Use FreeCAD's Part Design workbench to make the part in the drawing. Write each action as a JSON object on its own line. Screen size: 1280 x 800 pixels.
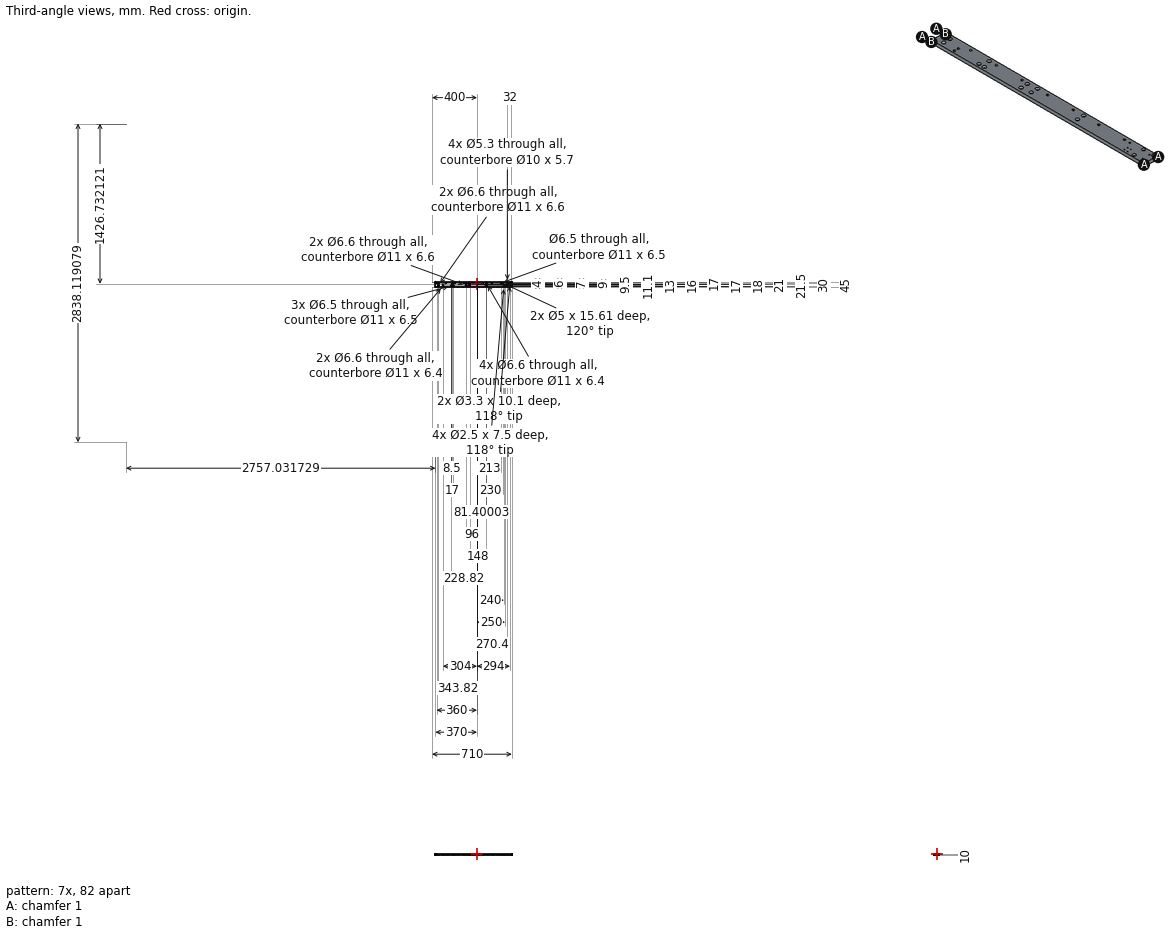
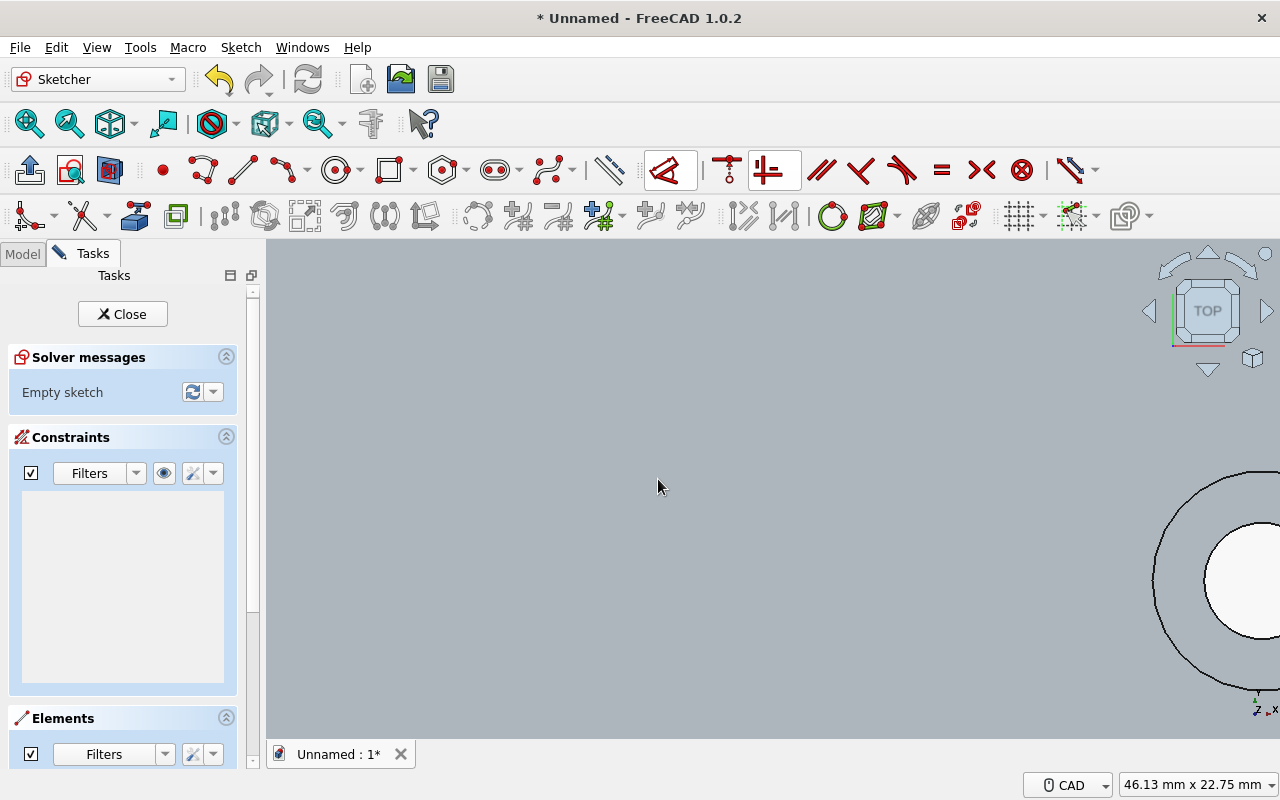
{"action": "left_click", "coordinate": [336, 170]}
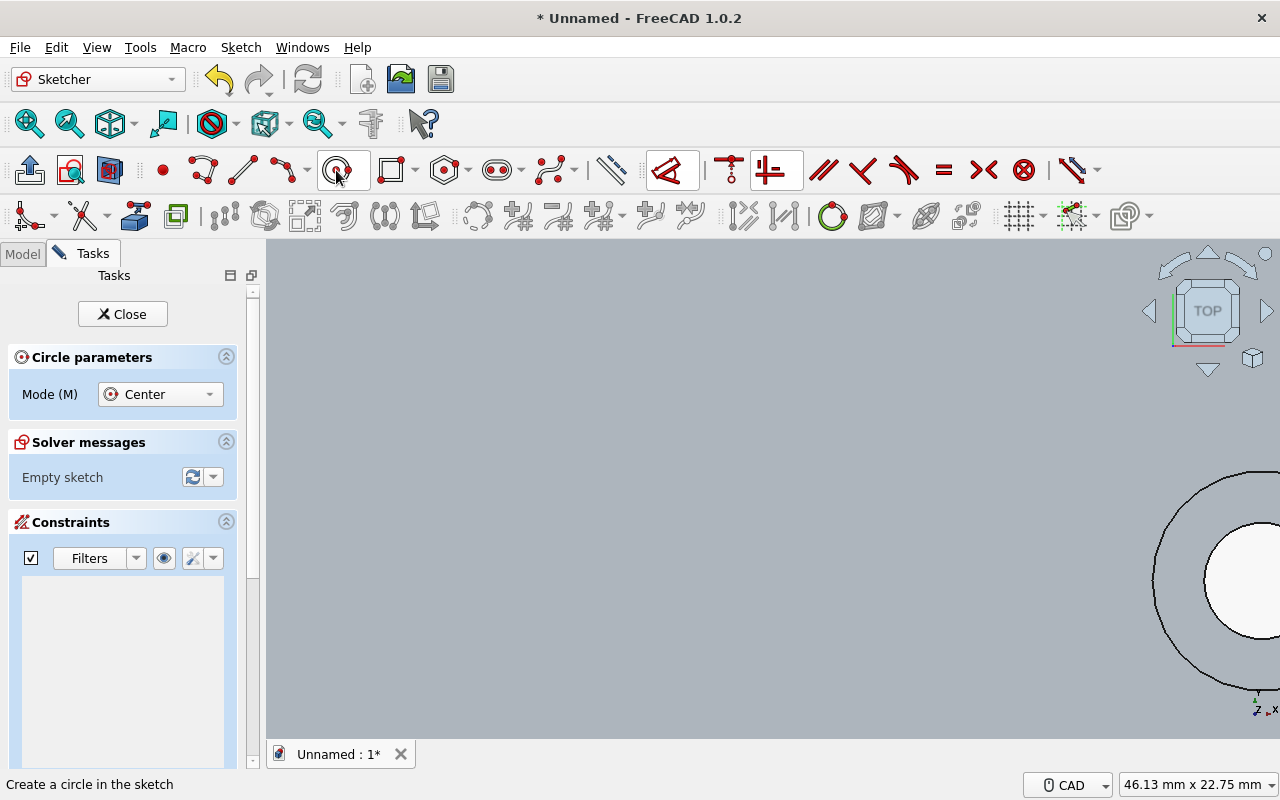
{"action": "left_click", "coordinate": [594, 603]}
{"action": "left_click", "coordinate": [614, 583]}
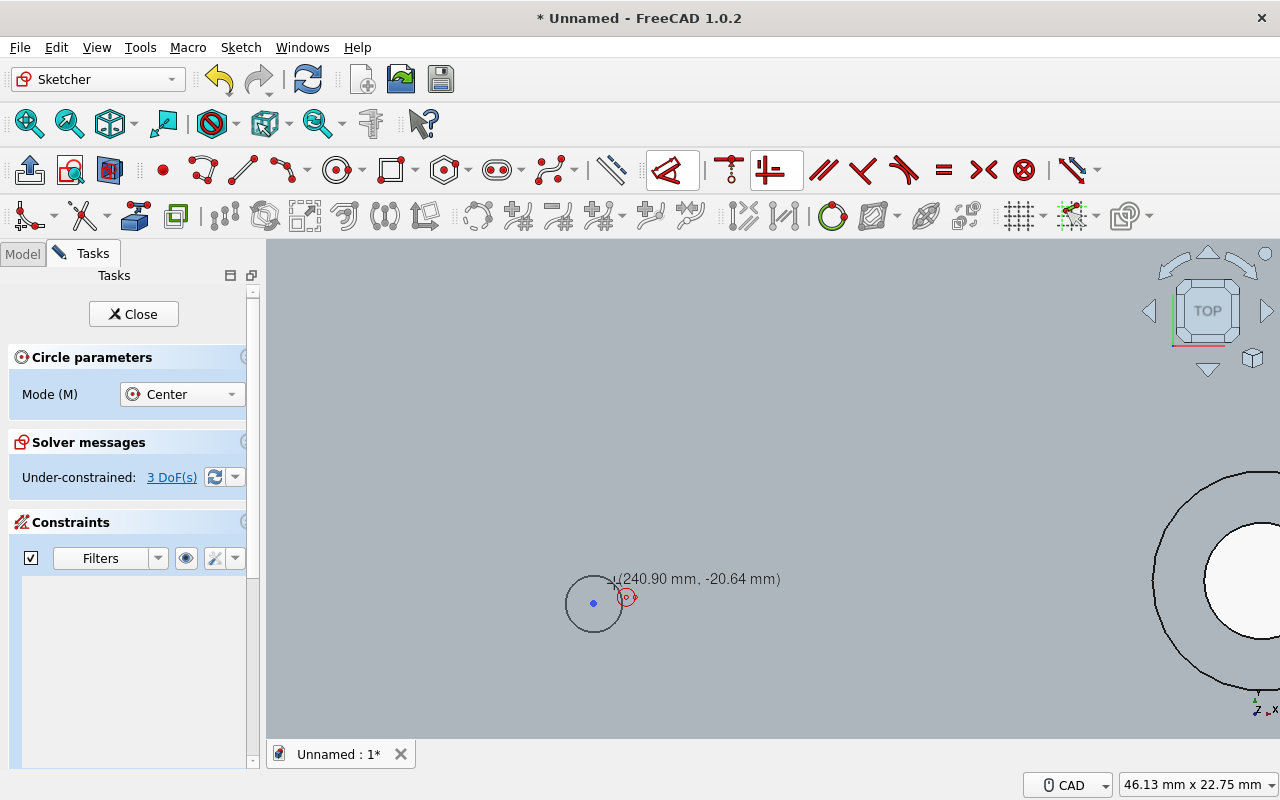
{"action": "left_click", "coordinate": [594, 374]}
{"action": "left_click", "coordinate": [614, 355]}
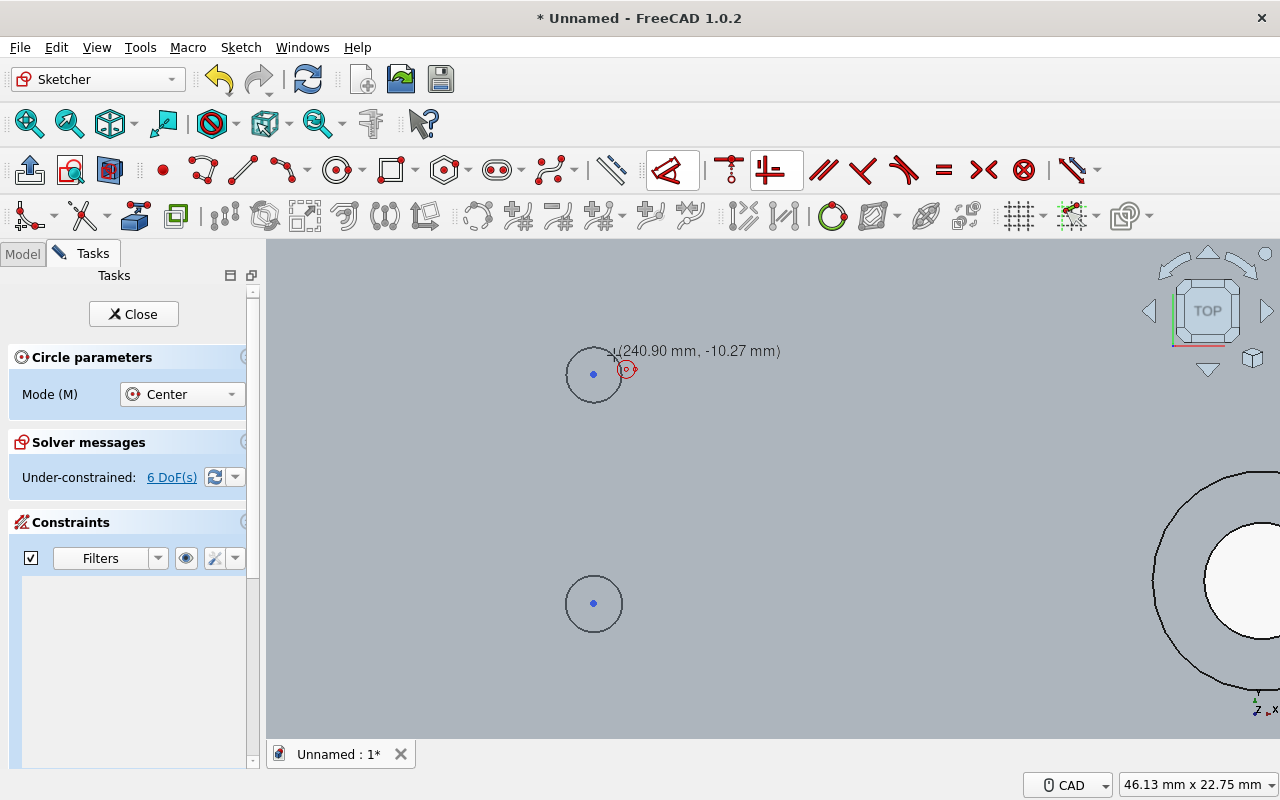
{"action": "left_click", "coordinate": [814, 374]}
{"action": "left_click", "coordinate": [833, 355]}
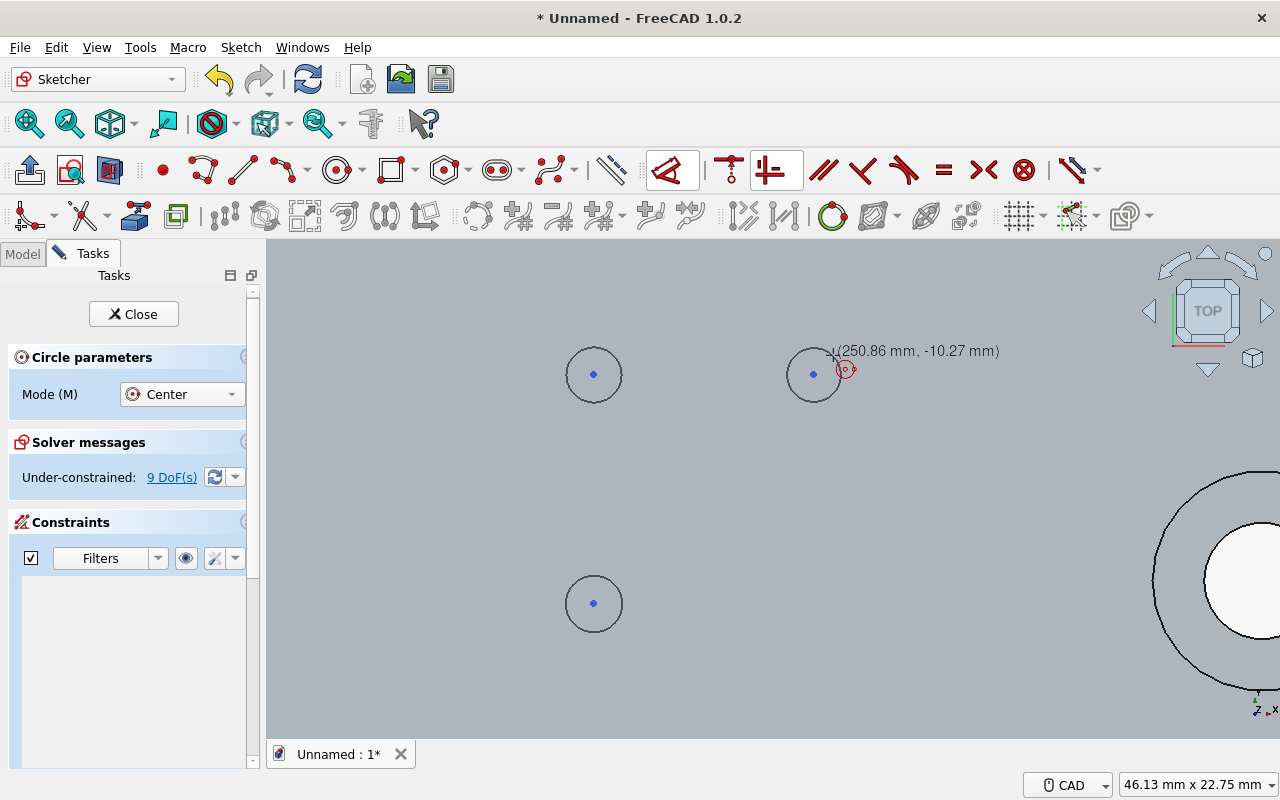
{"action": "left_click", "coordinate": [814, 603]}
{"action": "left_click", "coordinate": [833, 583]}
{"action": "key", "text": "Escape"}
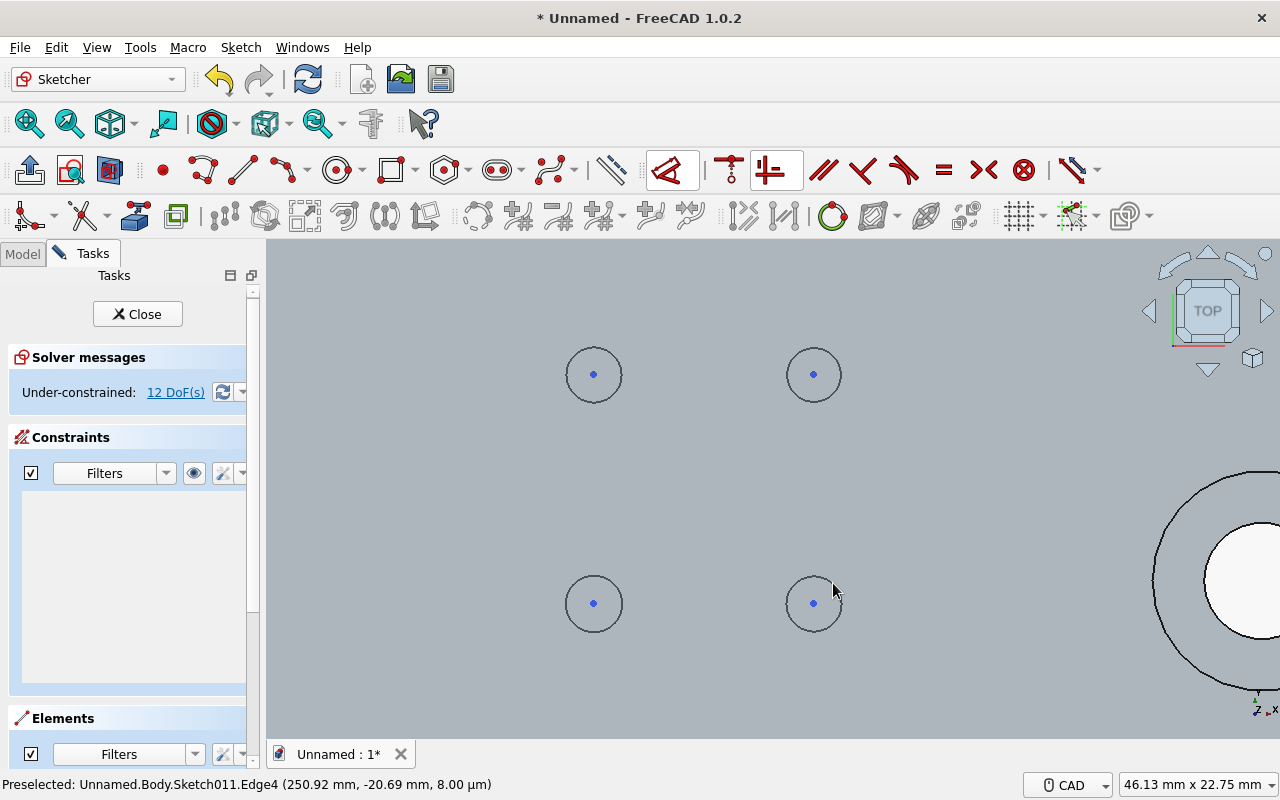
{"action": "left_click", "coordinate": [614, 584]}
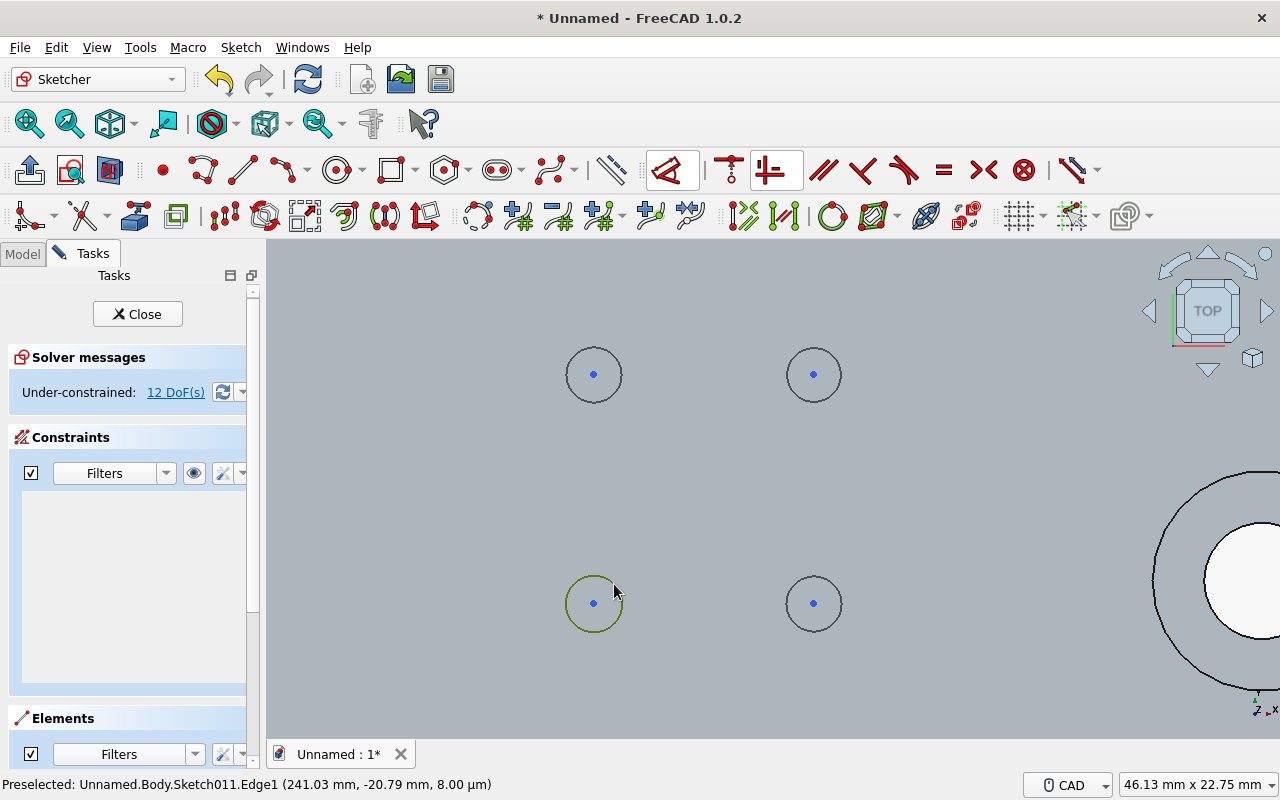
{"action": "left_click", "coordinate": [613, 355]}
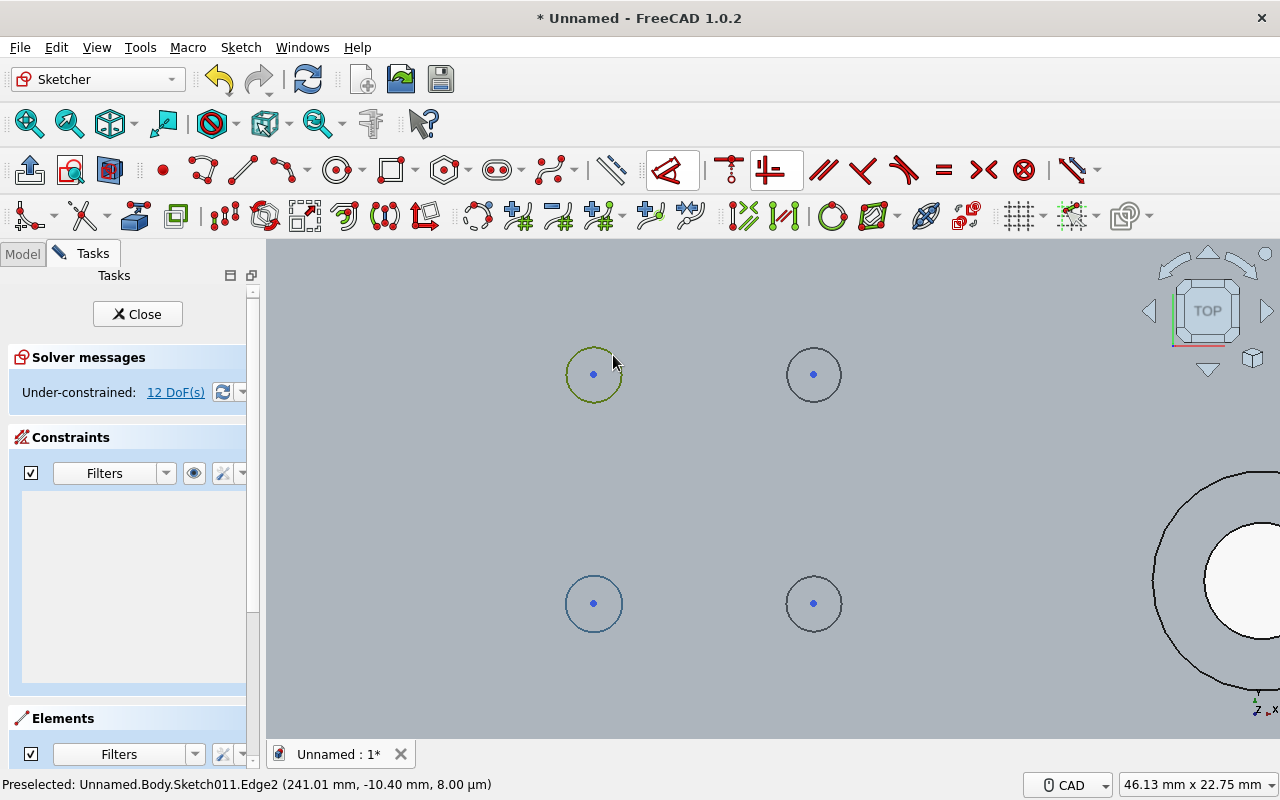
{"action": "left_click", "coordinate": [833, 356]}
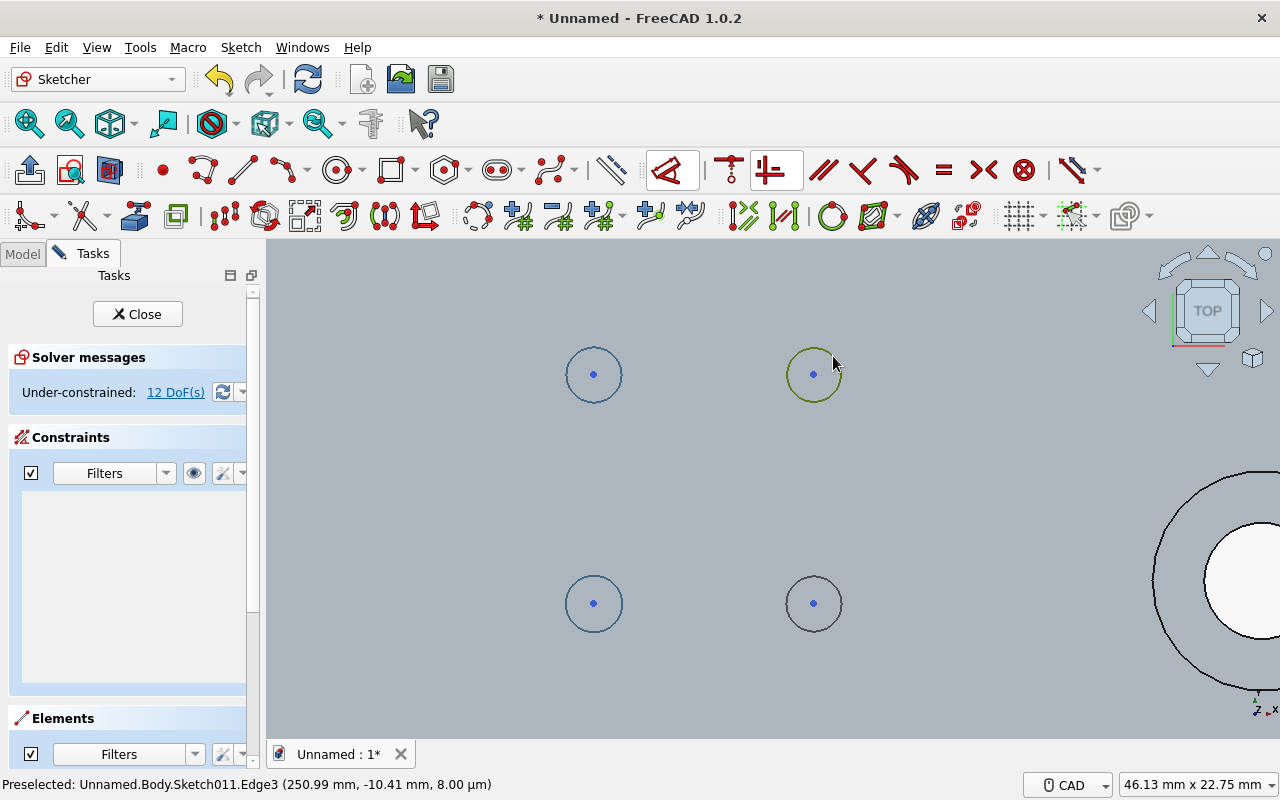
{"action": "left_click", "coordinate": [833, 584]}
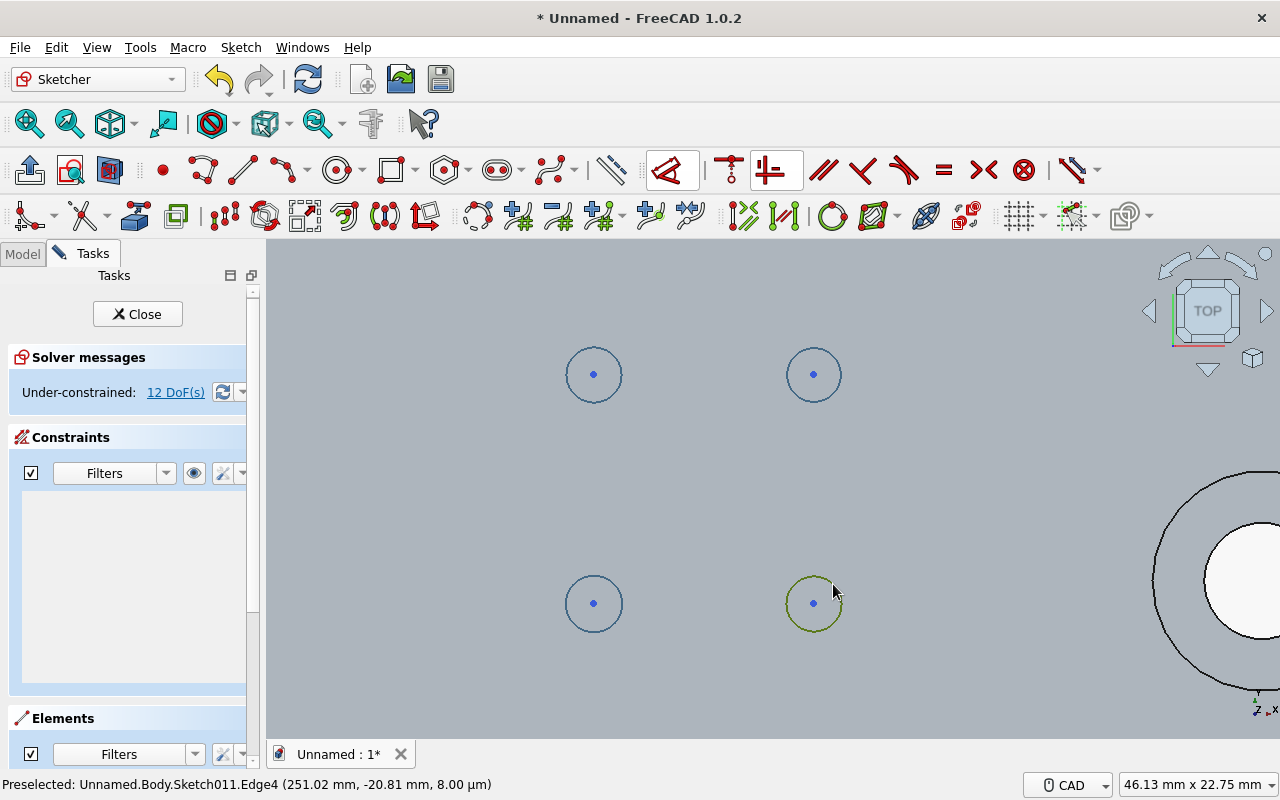
{"action": "left_click", "coordinate": [944, 170]}